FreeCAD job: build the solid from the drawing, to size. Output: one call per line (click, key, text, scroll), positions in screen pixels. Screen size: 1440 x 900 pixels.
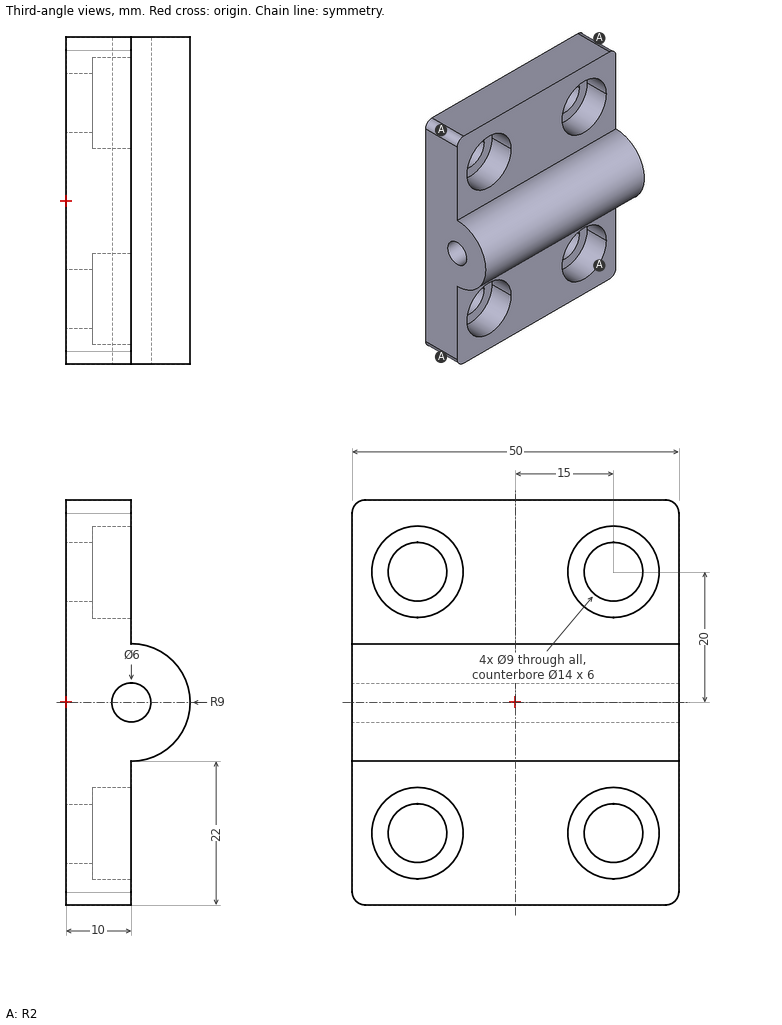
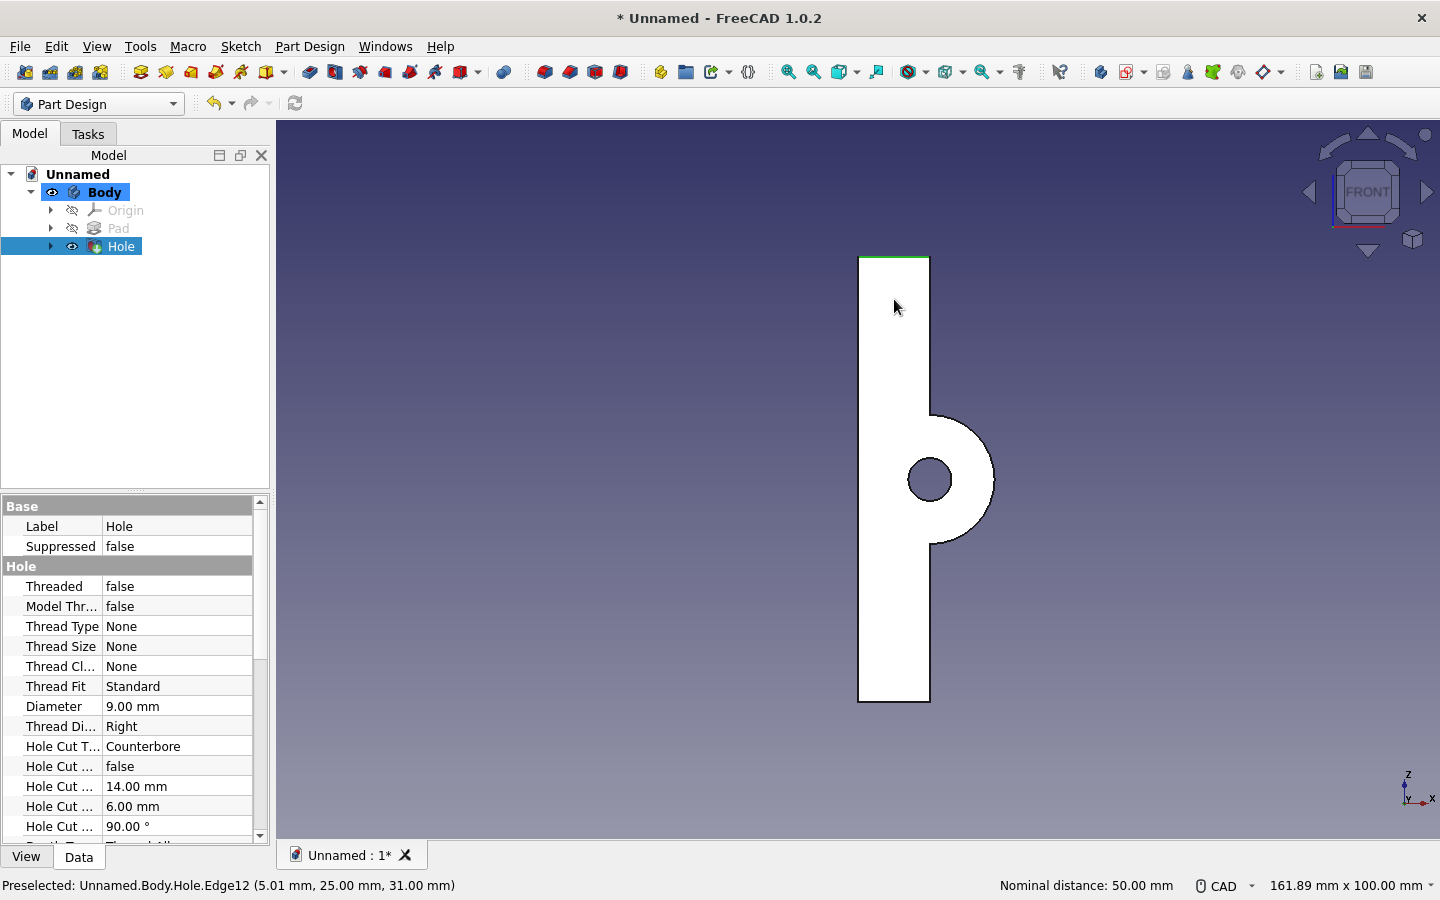
key(3)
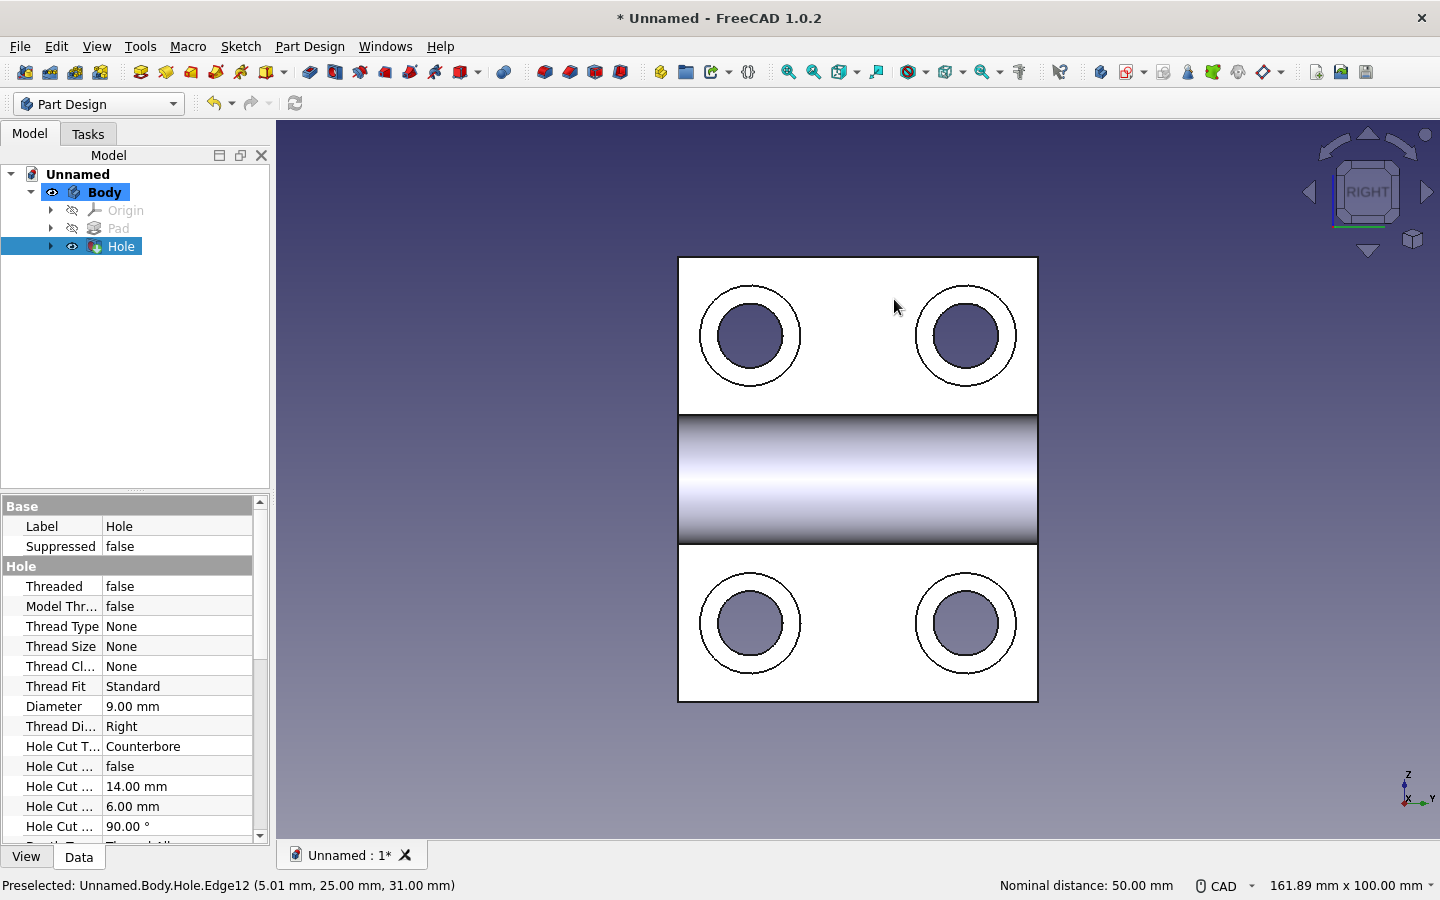
key(5)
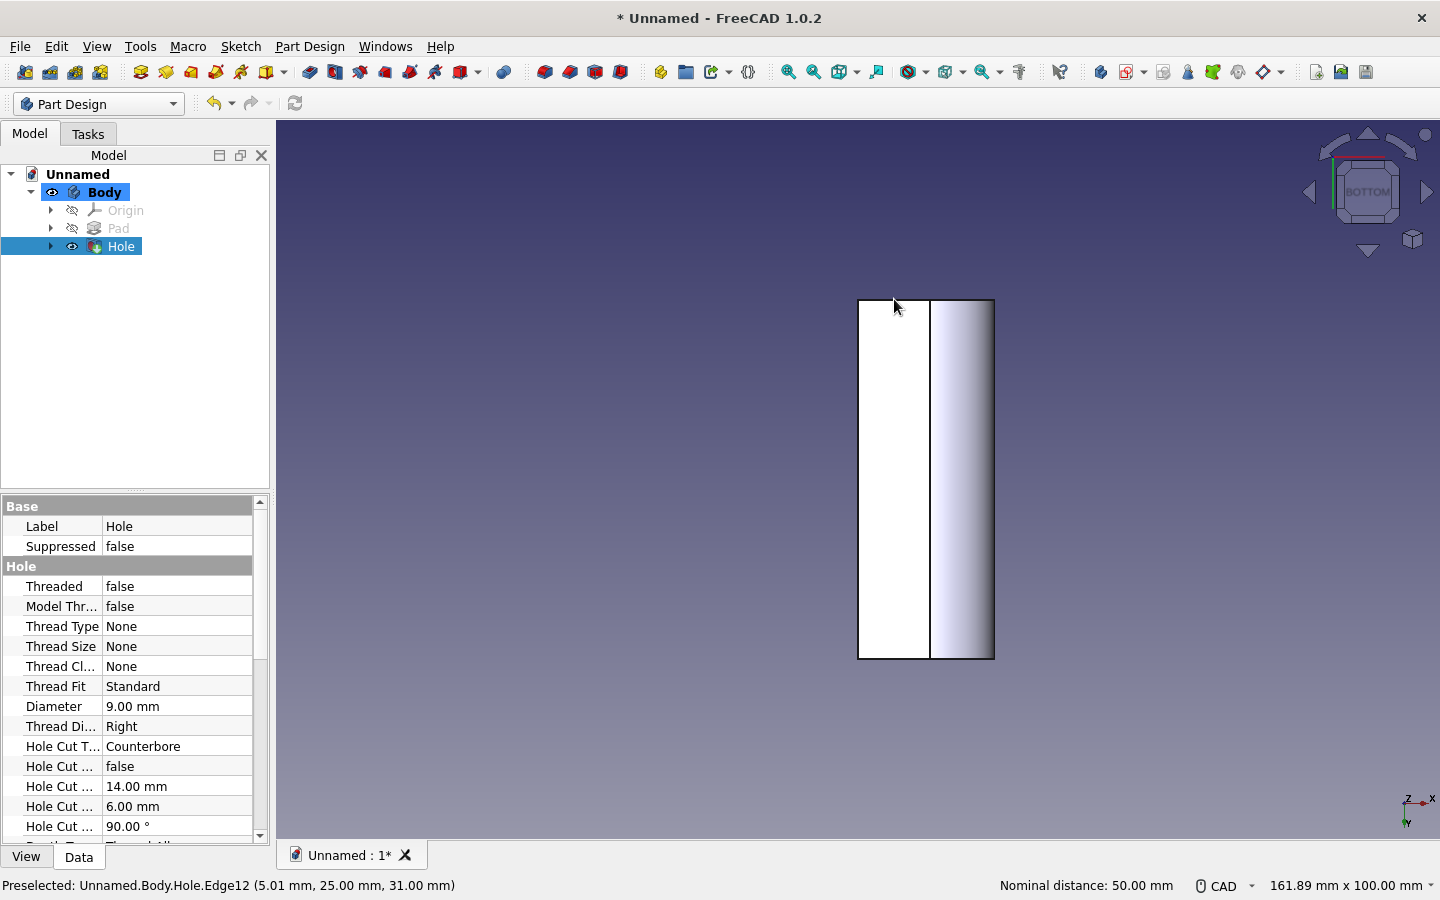
click(894, 299, ctrl)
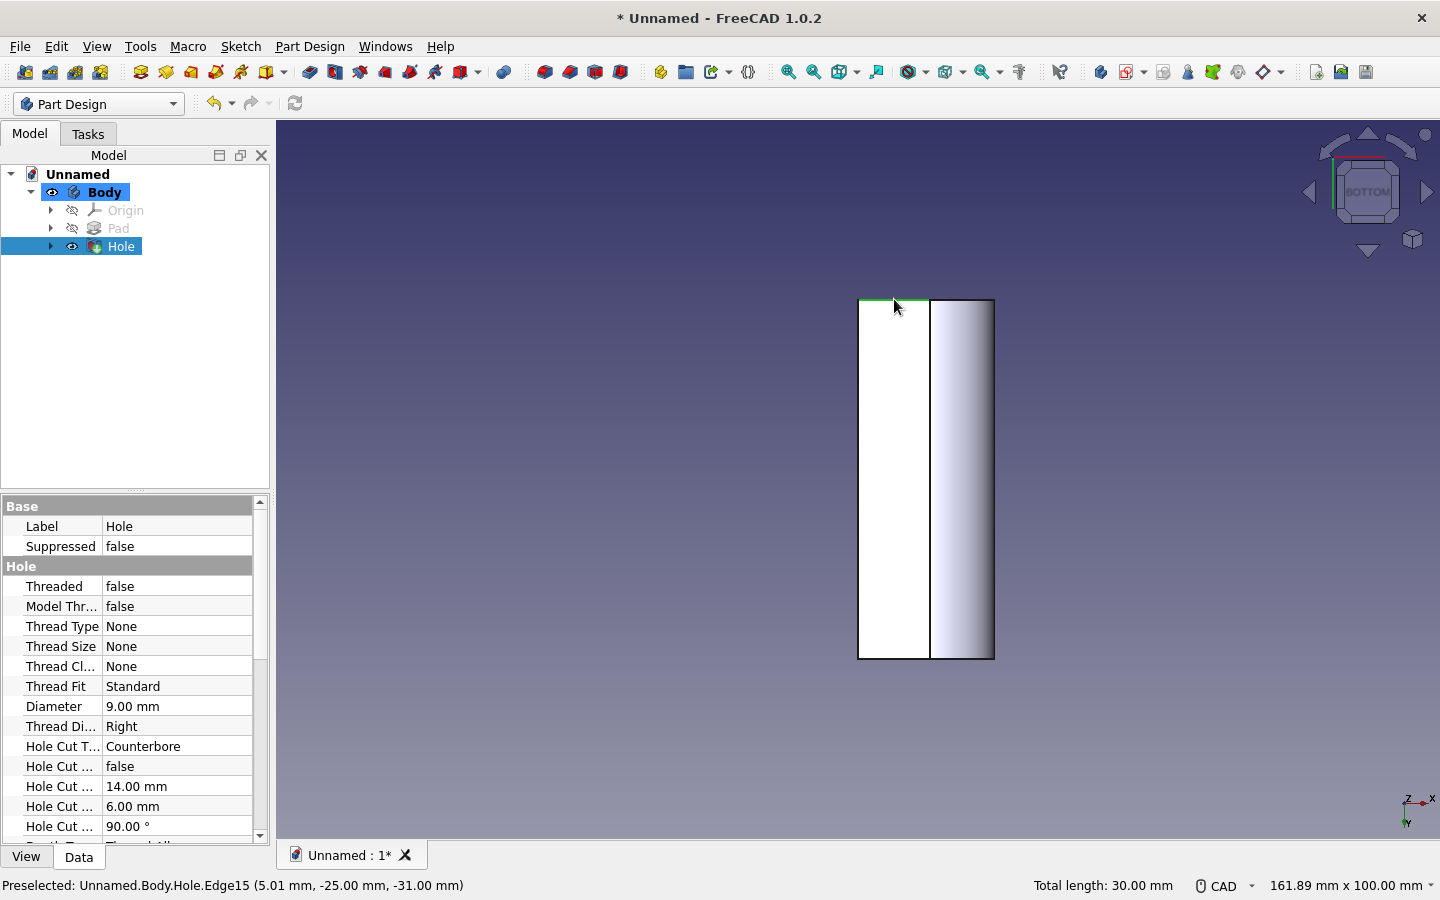
key(4)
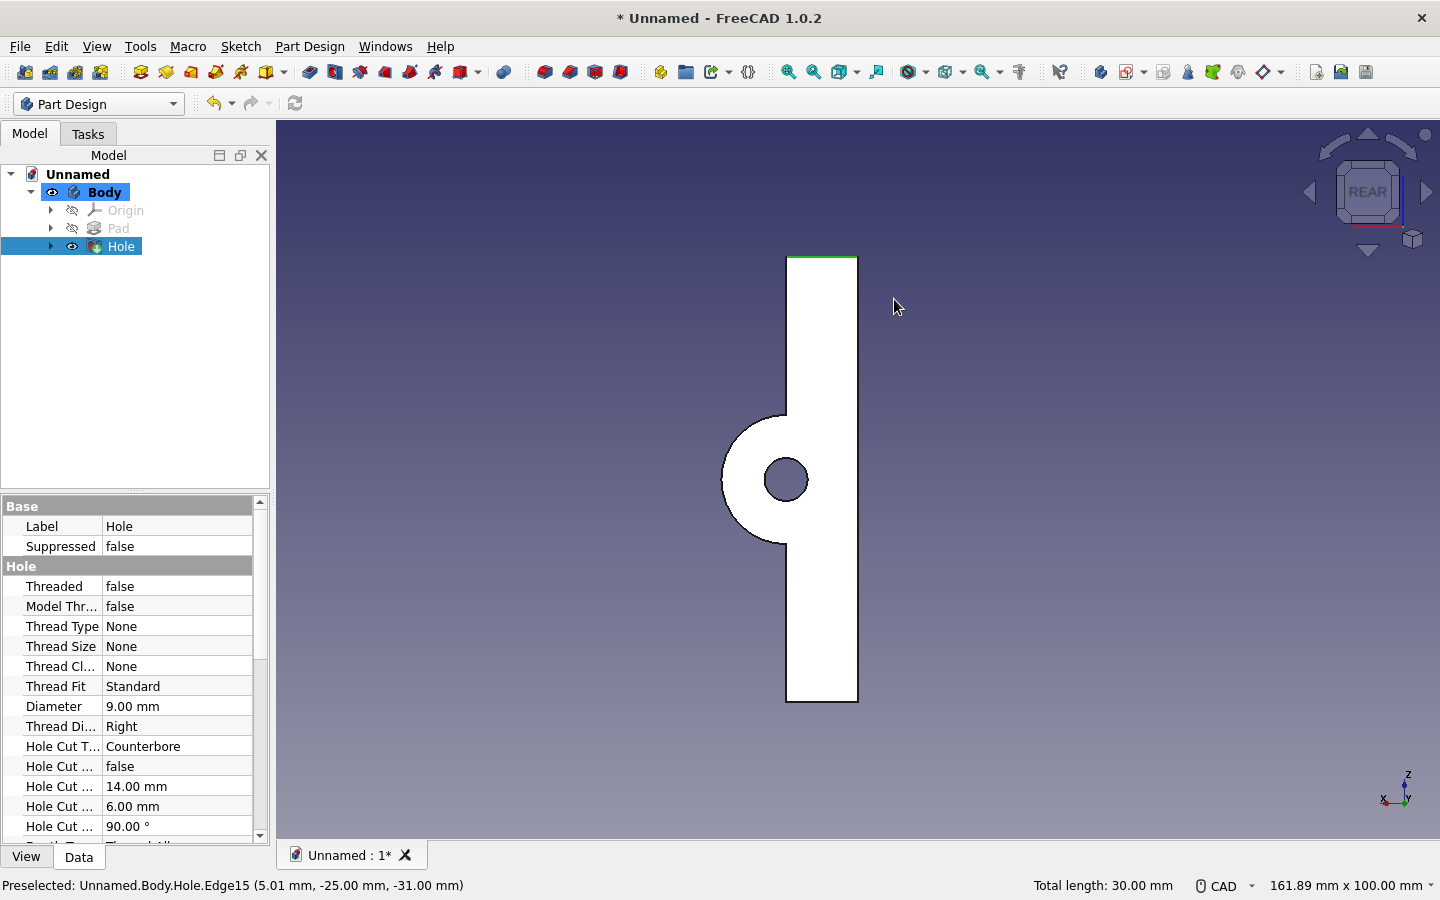
click(822, 701, ctrl)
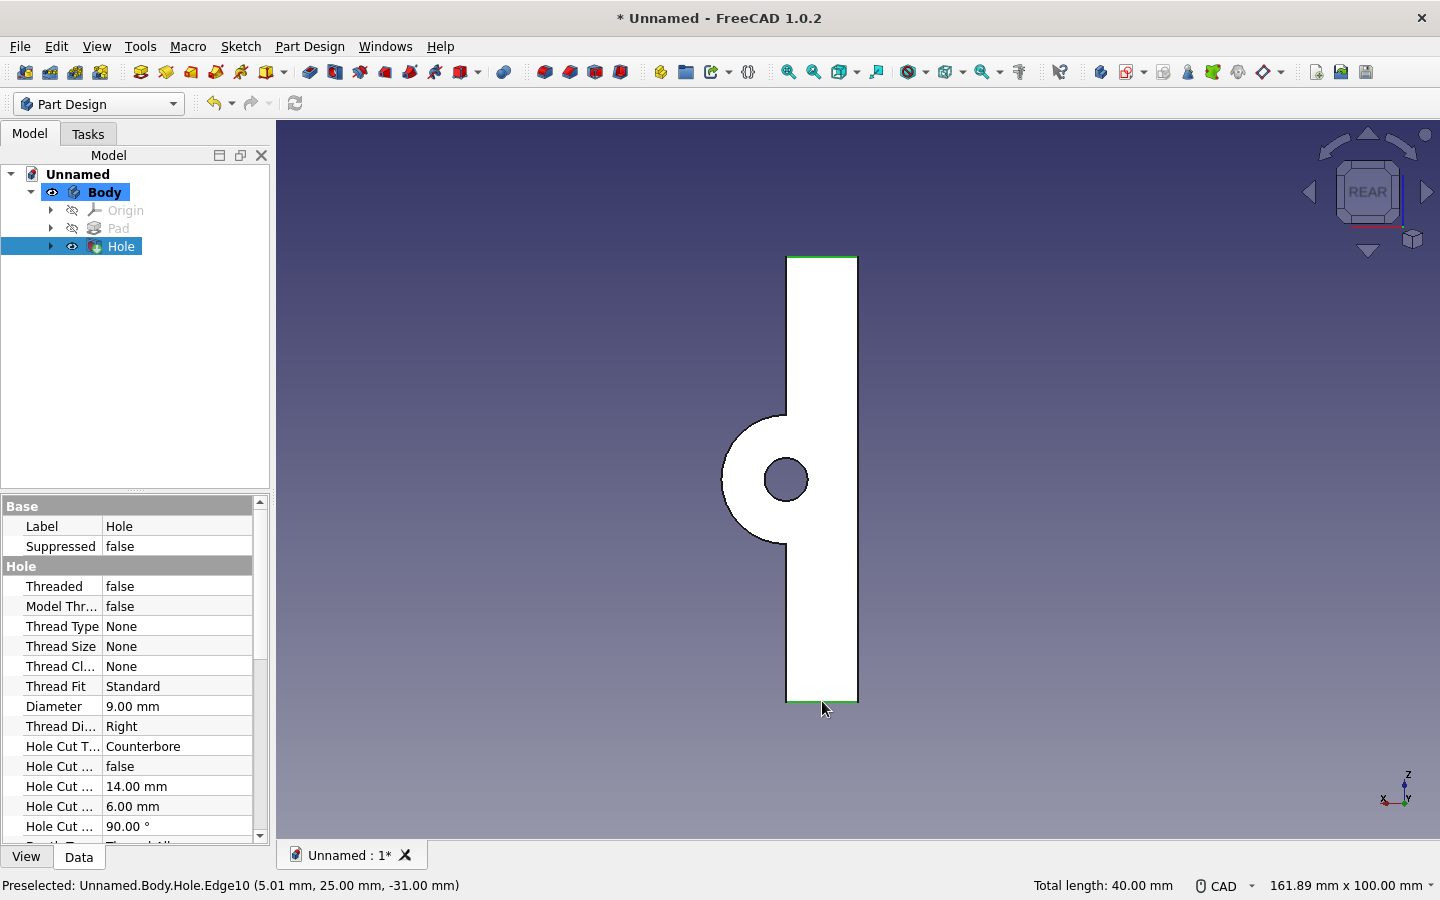
click(545, 72)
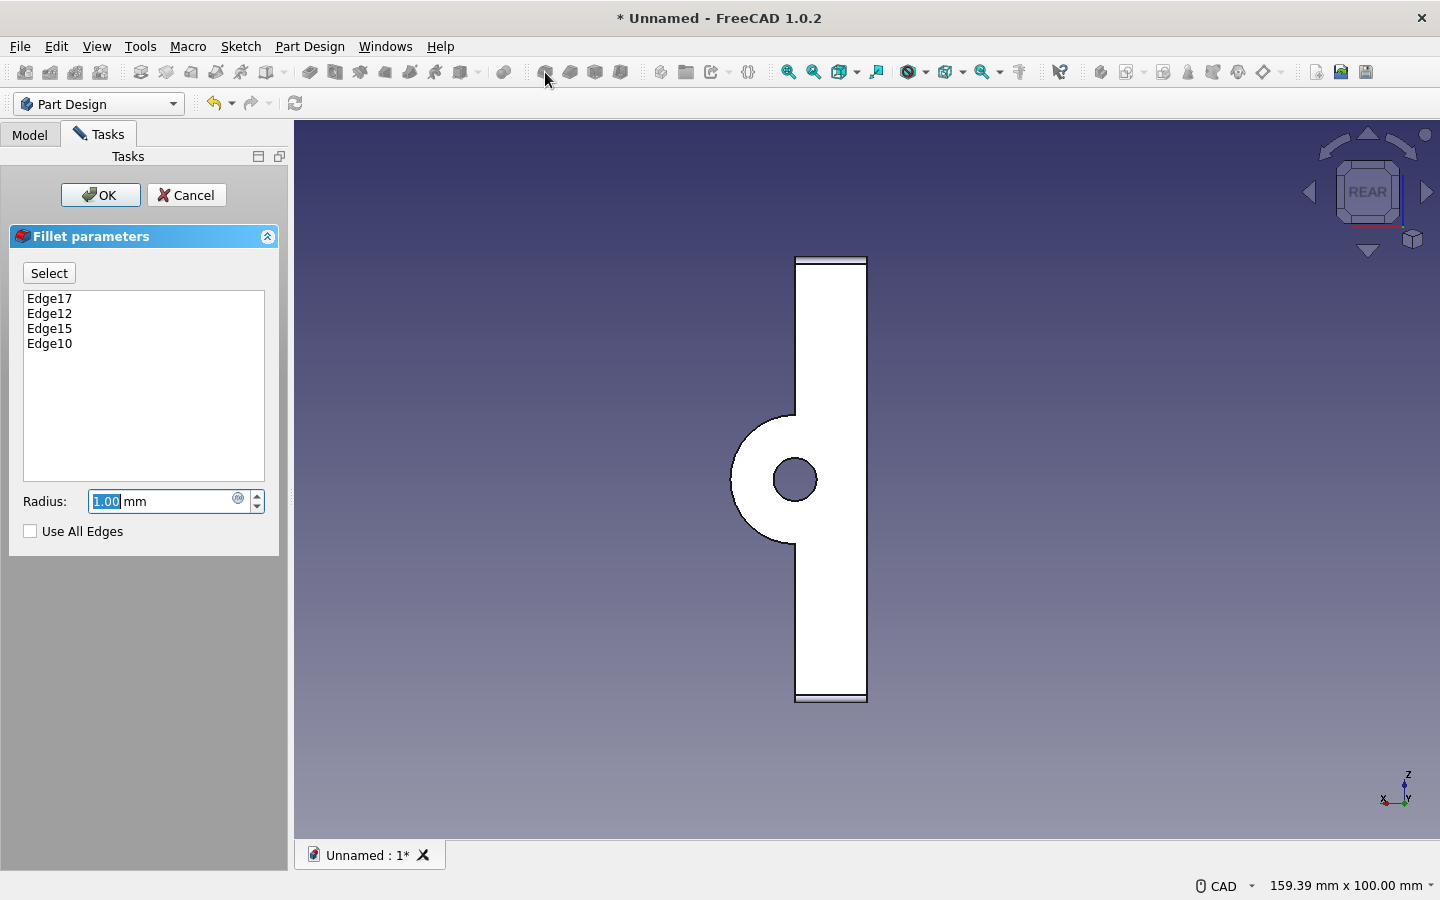
text(2)
key(Tab)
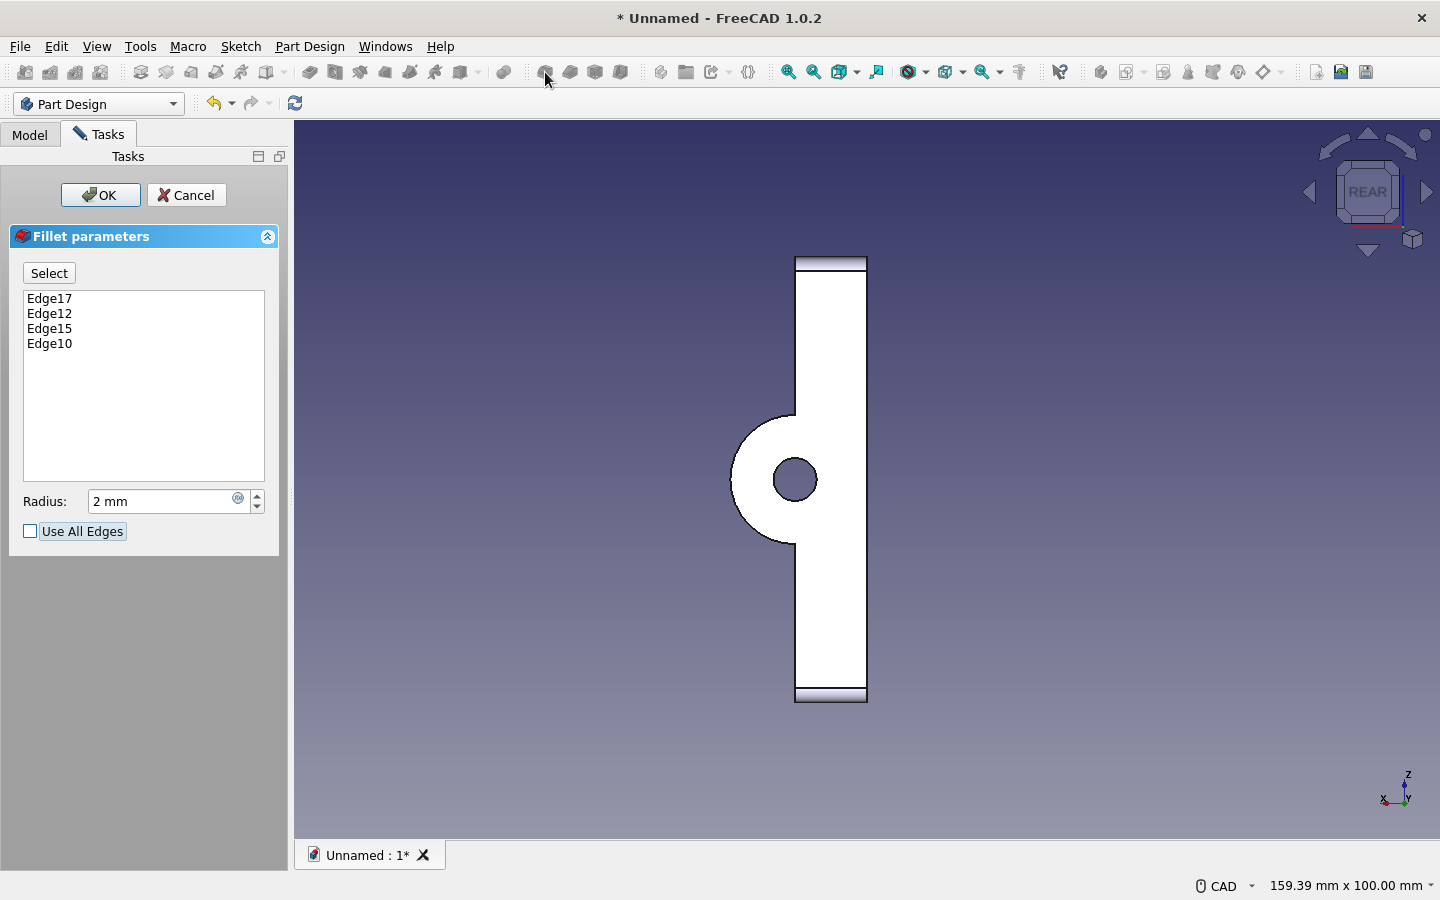
click(101, 195)